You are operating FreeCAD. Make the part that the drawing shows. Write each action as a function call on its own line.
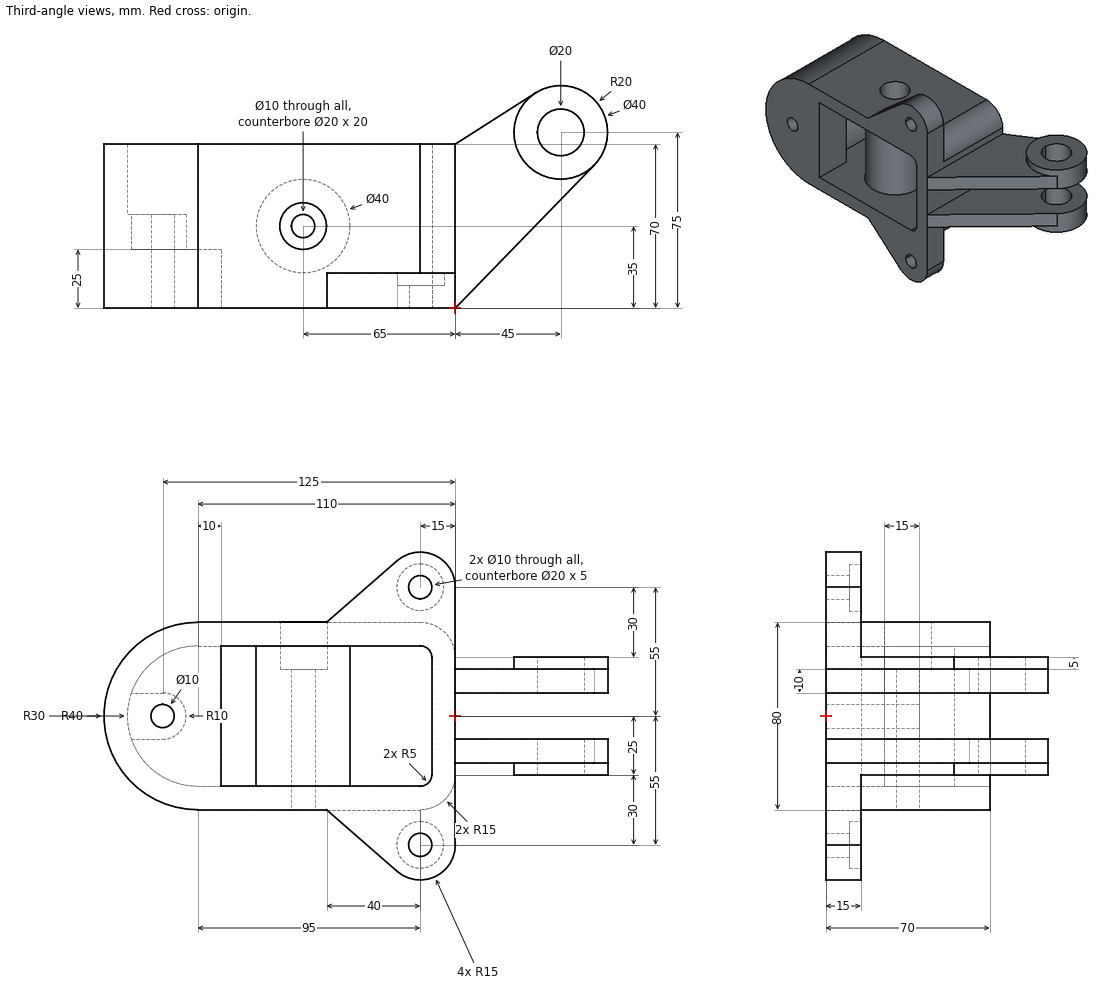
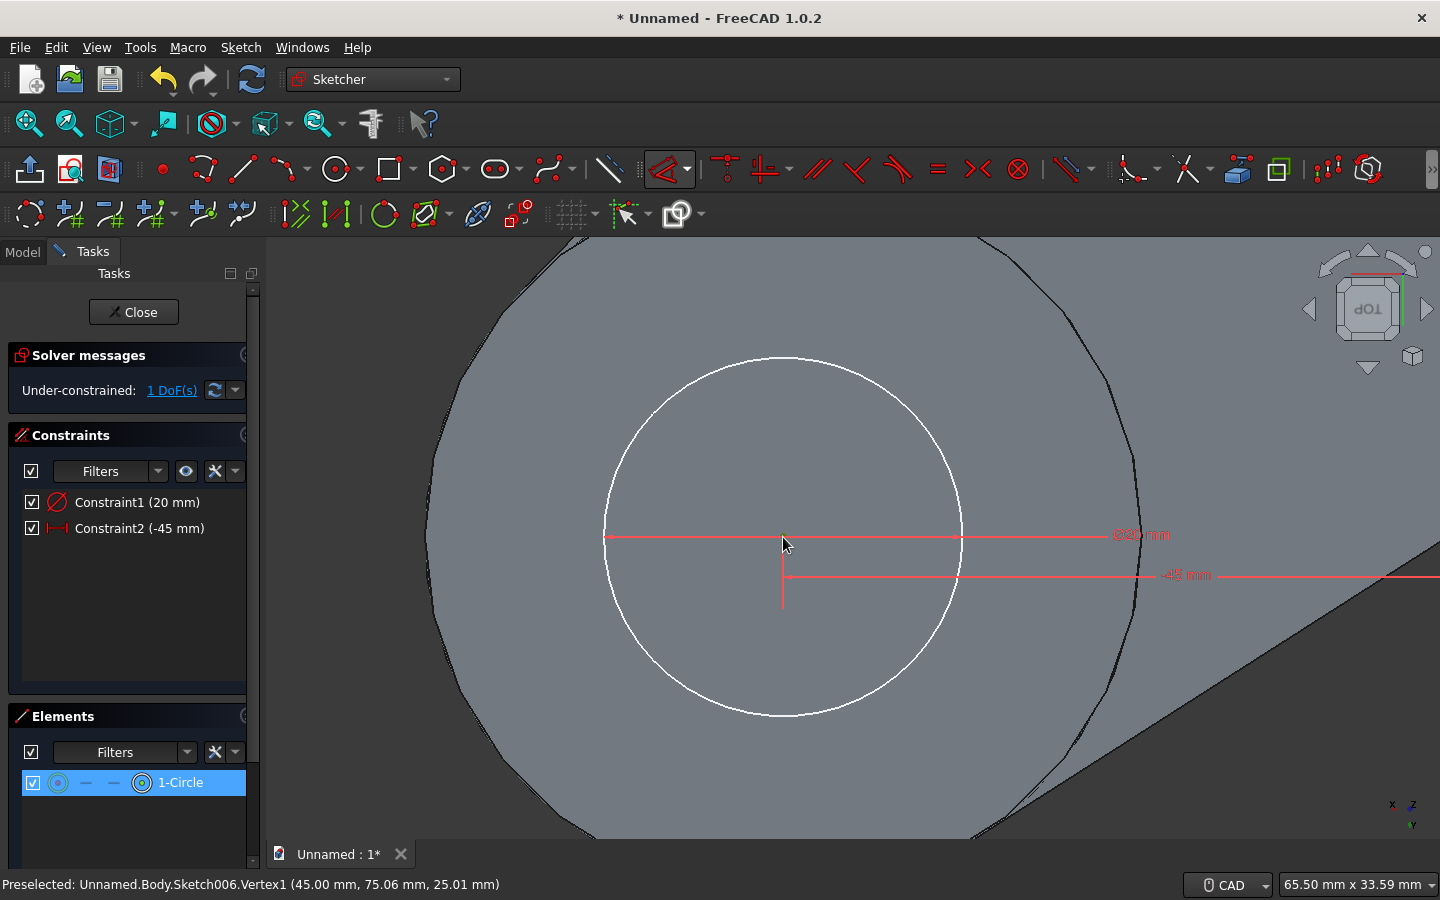
key(i)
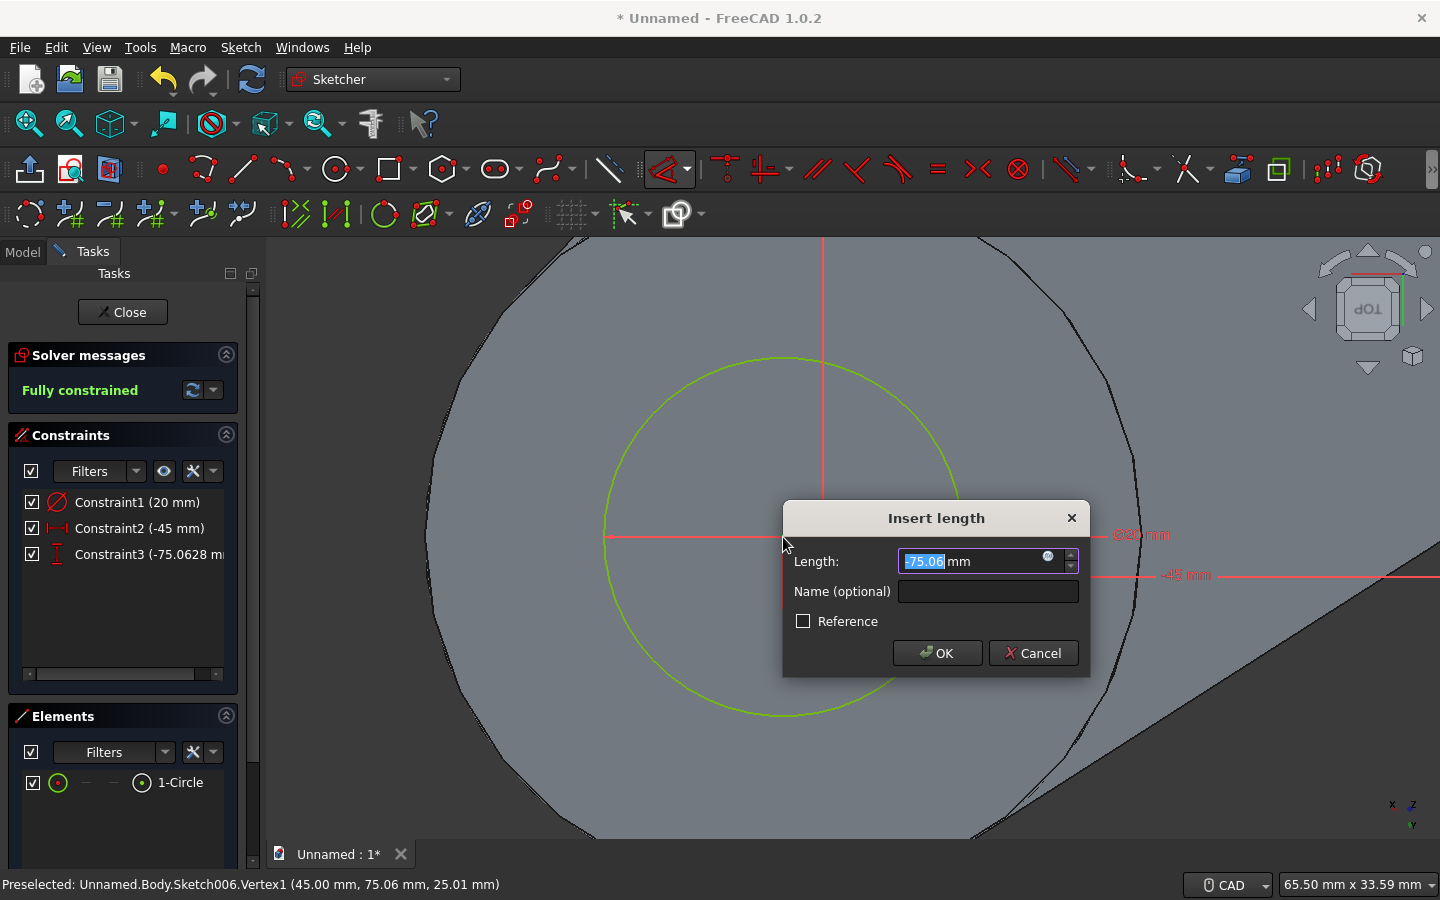
text(-75)
key(Return)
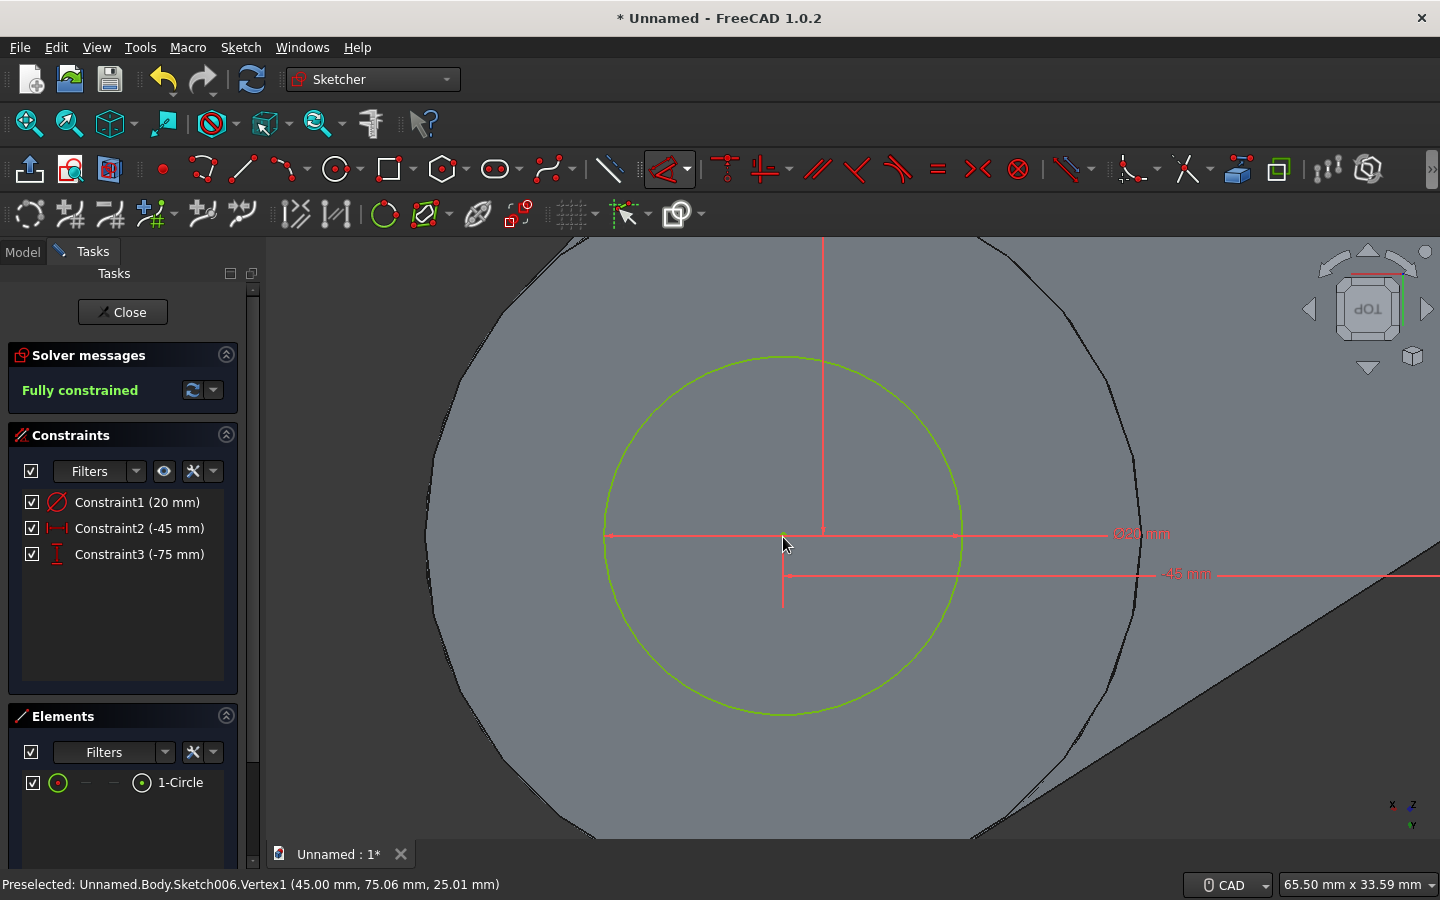
click(123, 312)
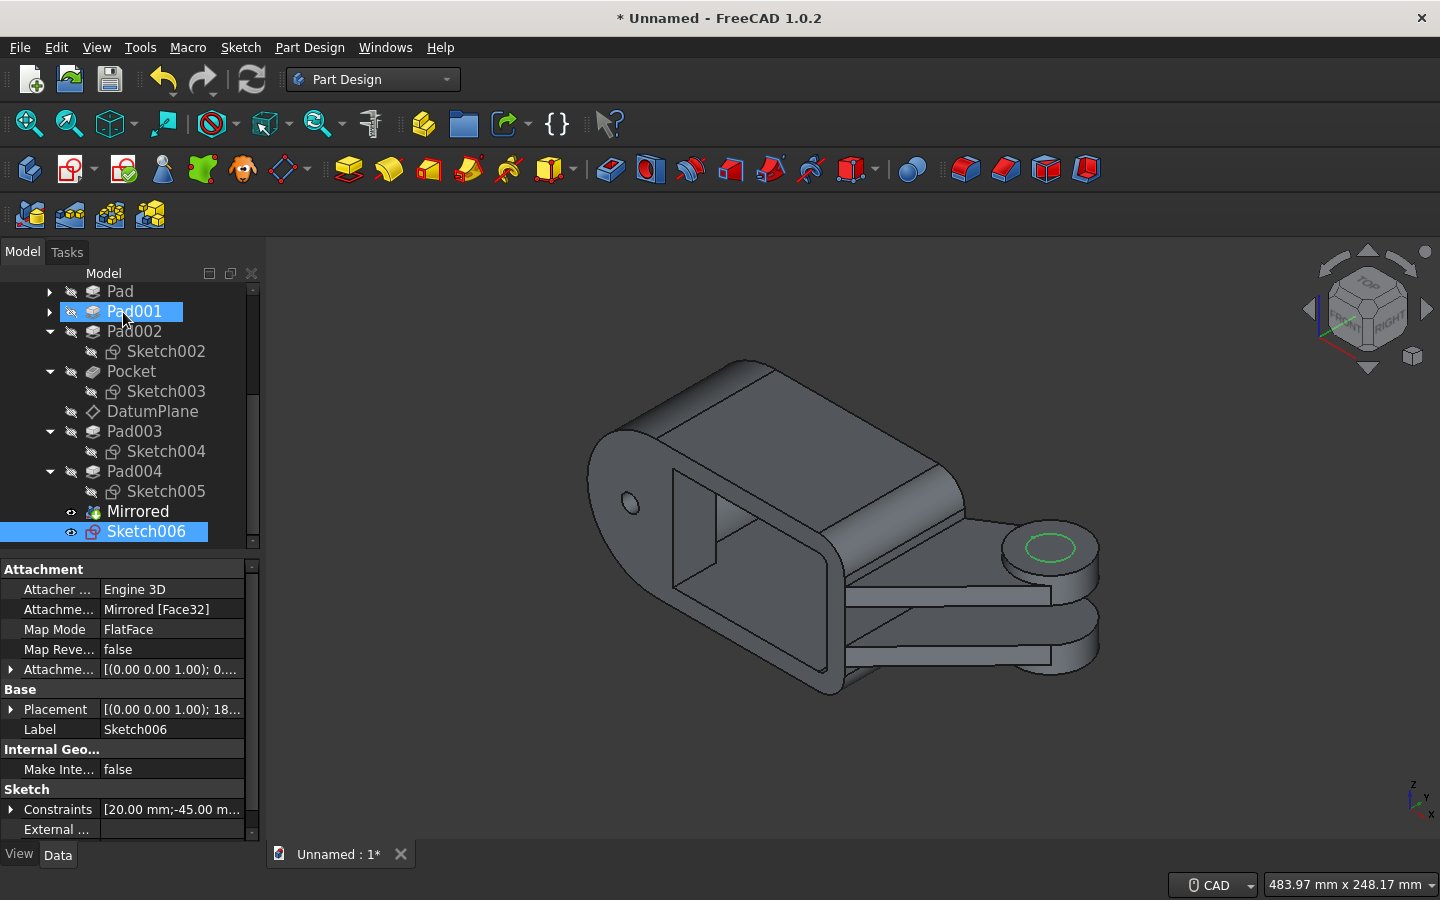
click(612, 170)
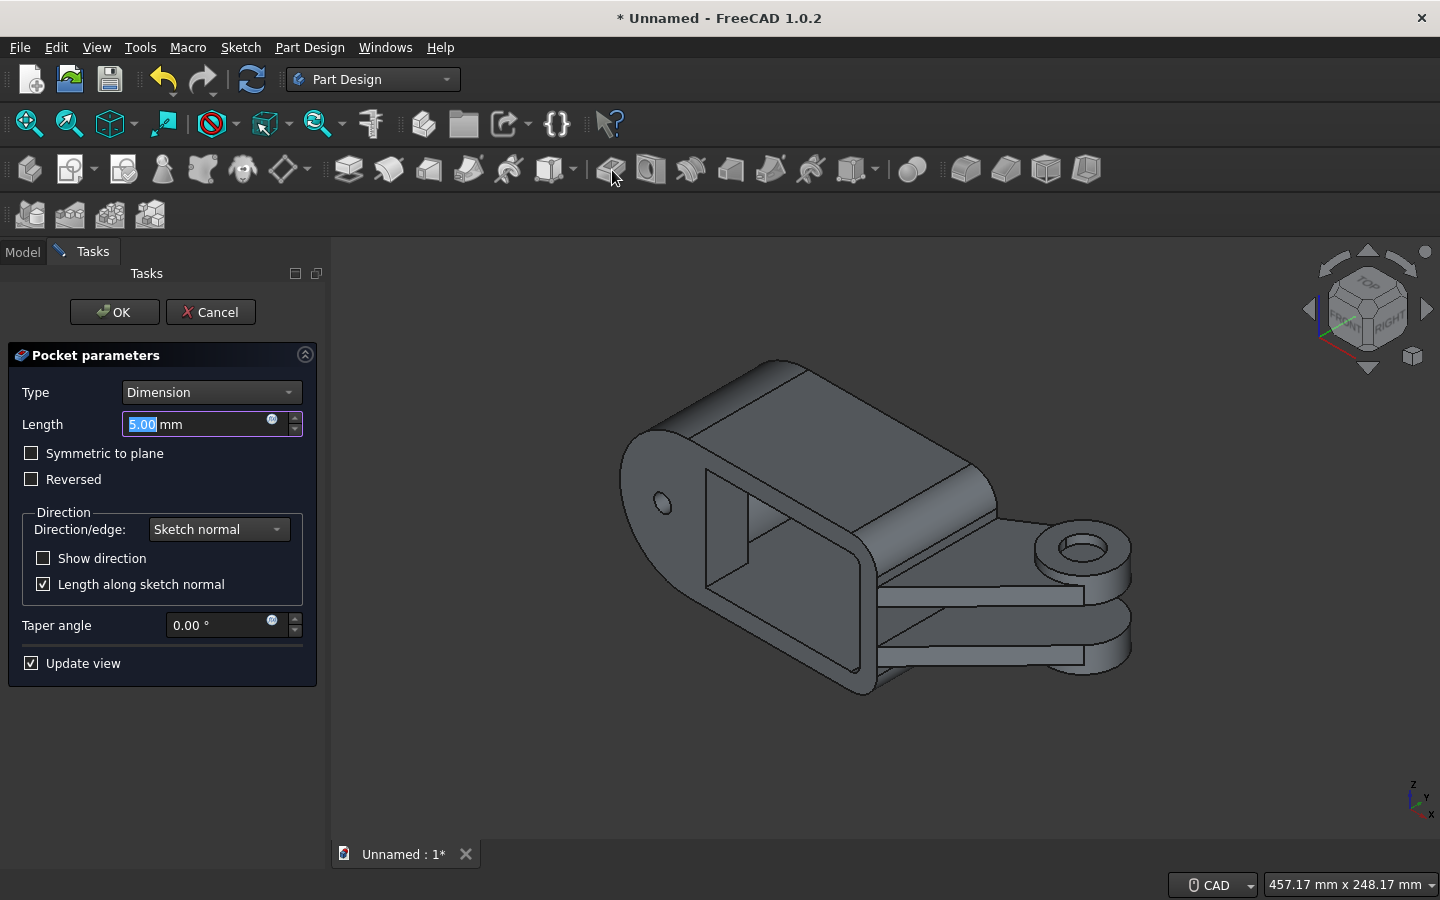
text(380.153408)
key(Tab)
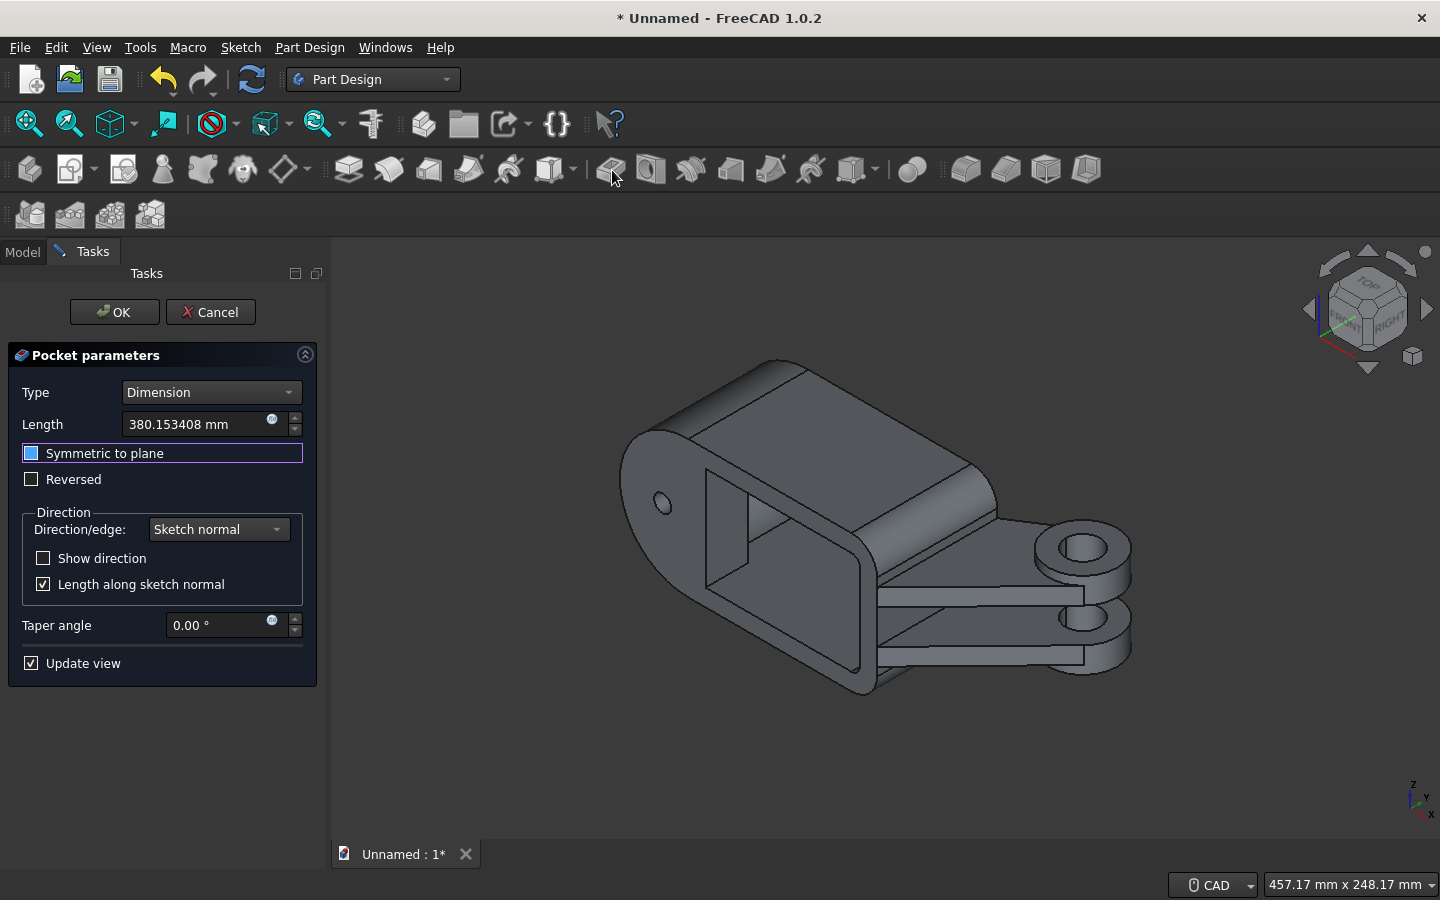
click(30, 453)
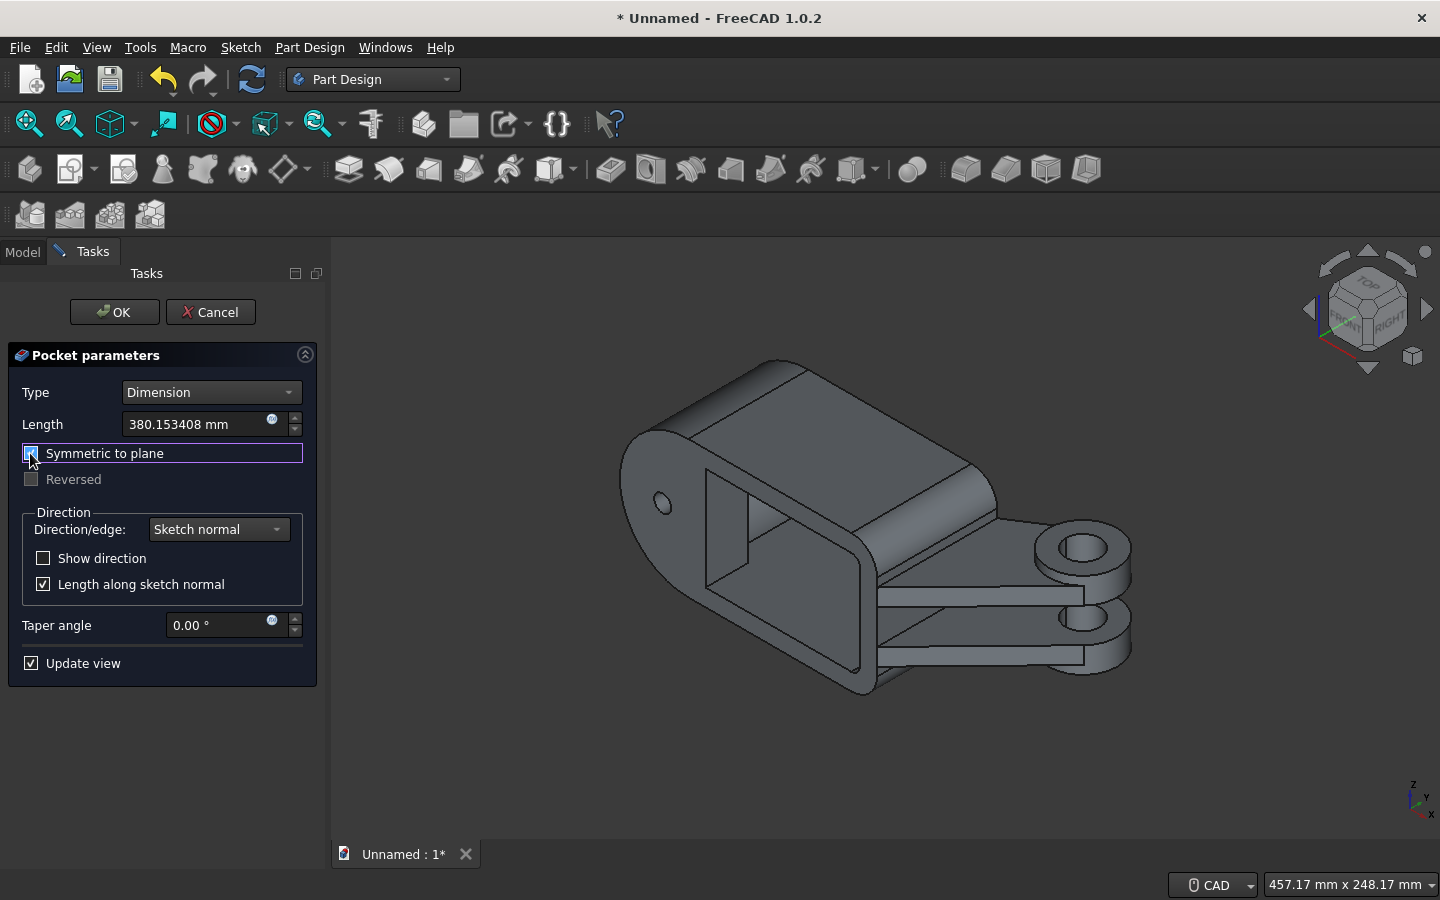
click(115, 312)